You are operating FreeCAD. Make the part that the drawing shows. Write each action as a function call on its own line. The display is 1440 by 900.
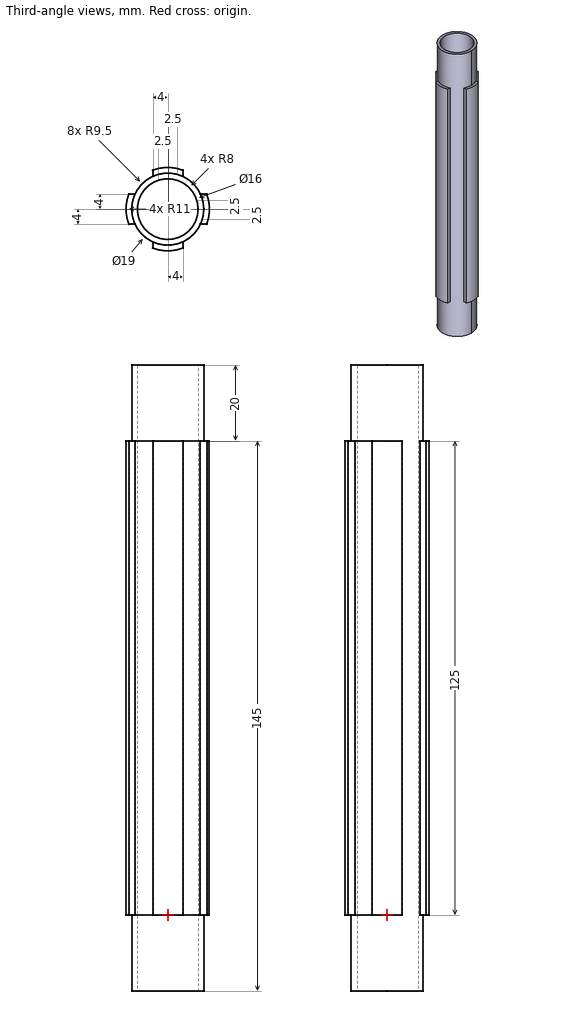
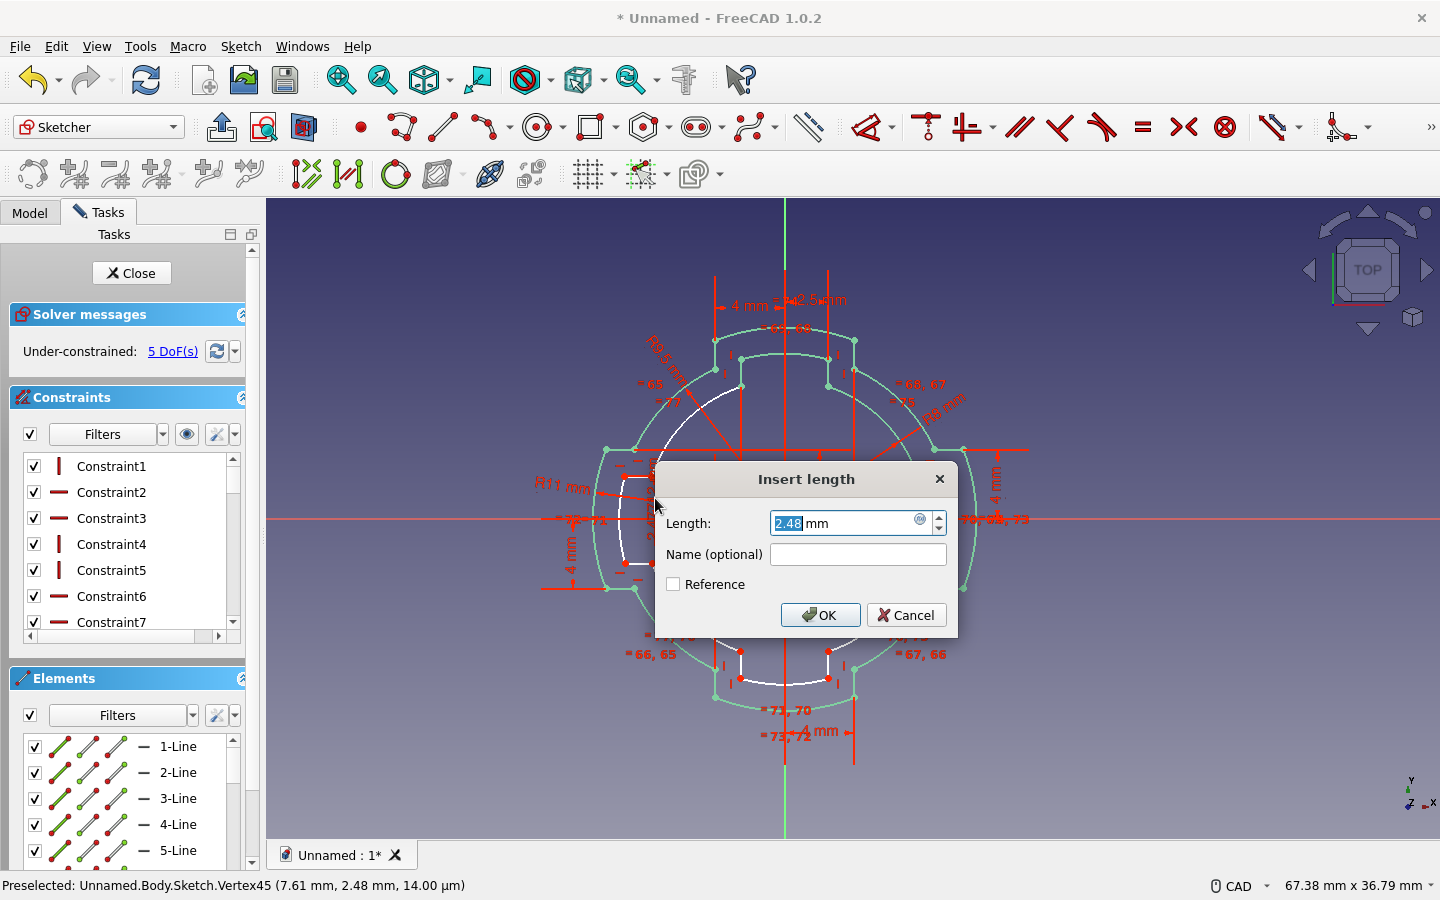
text(2.5)
key(Return)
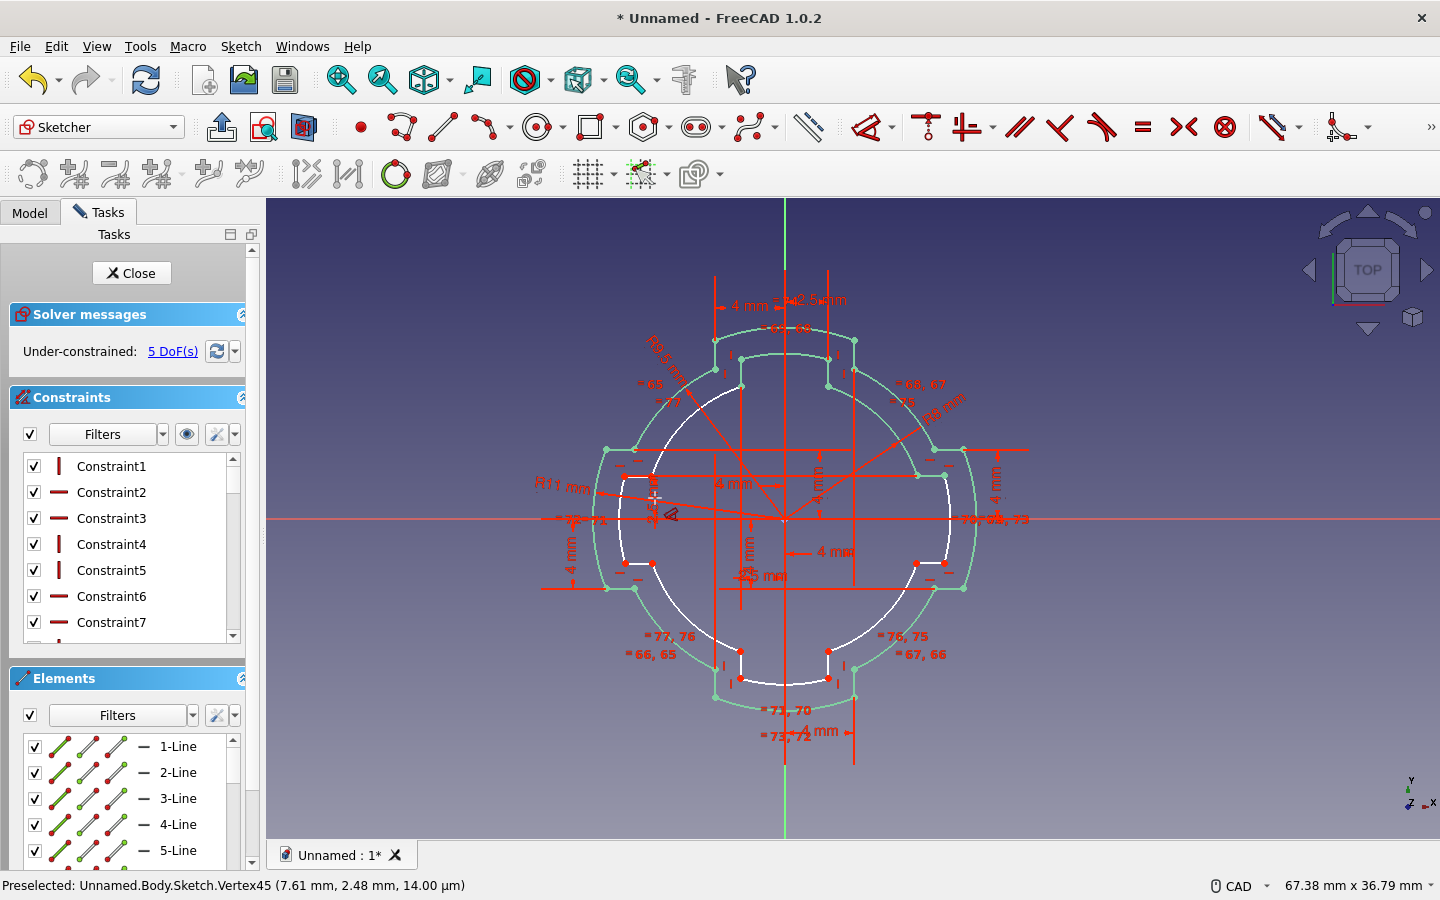
click(944, 563)
click(1002, 541)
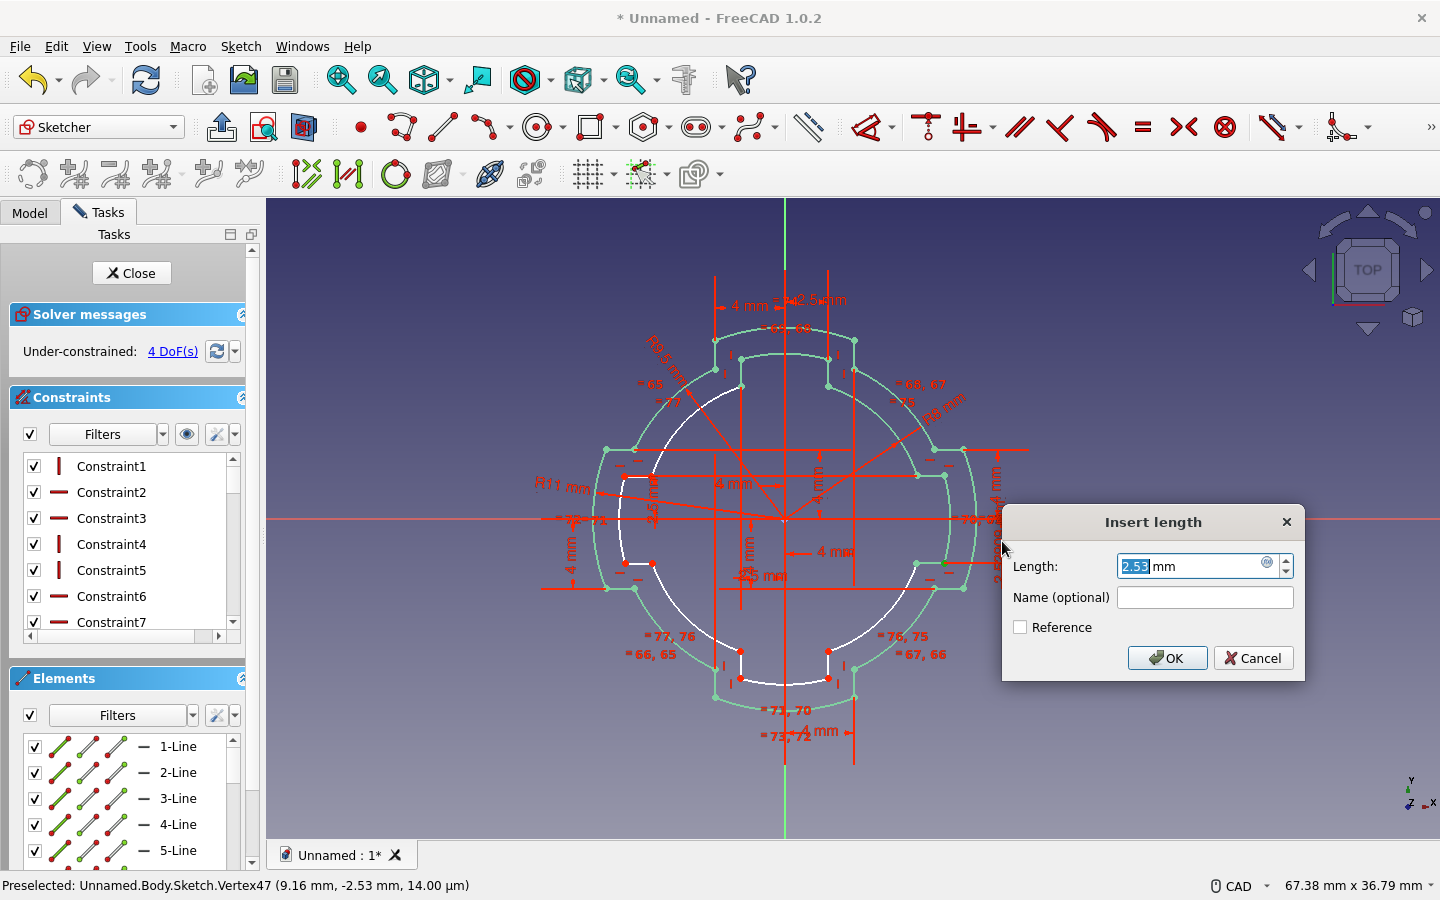
text(2.5)
key(Return)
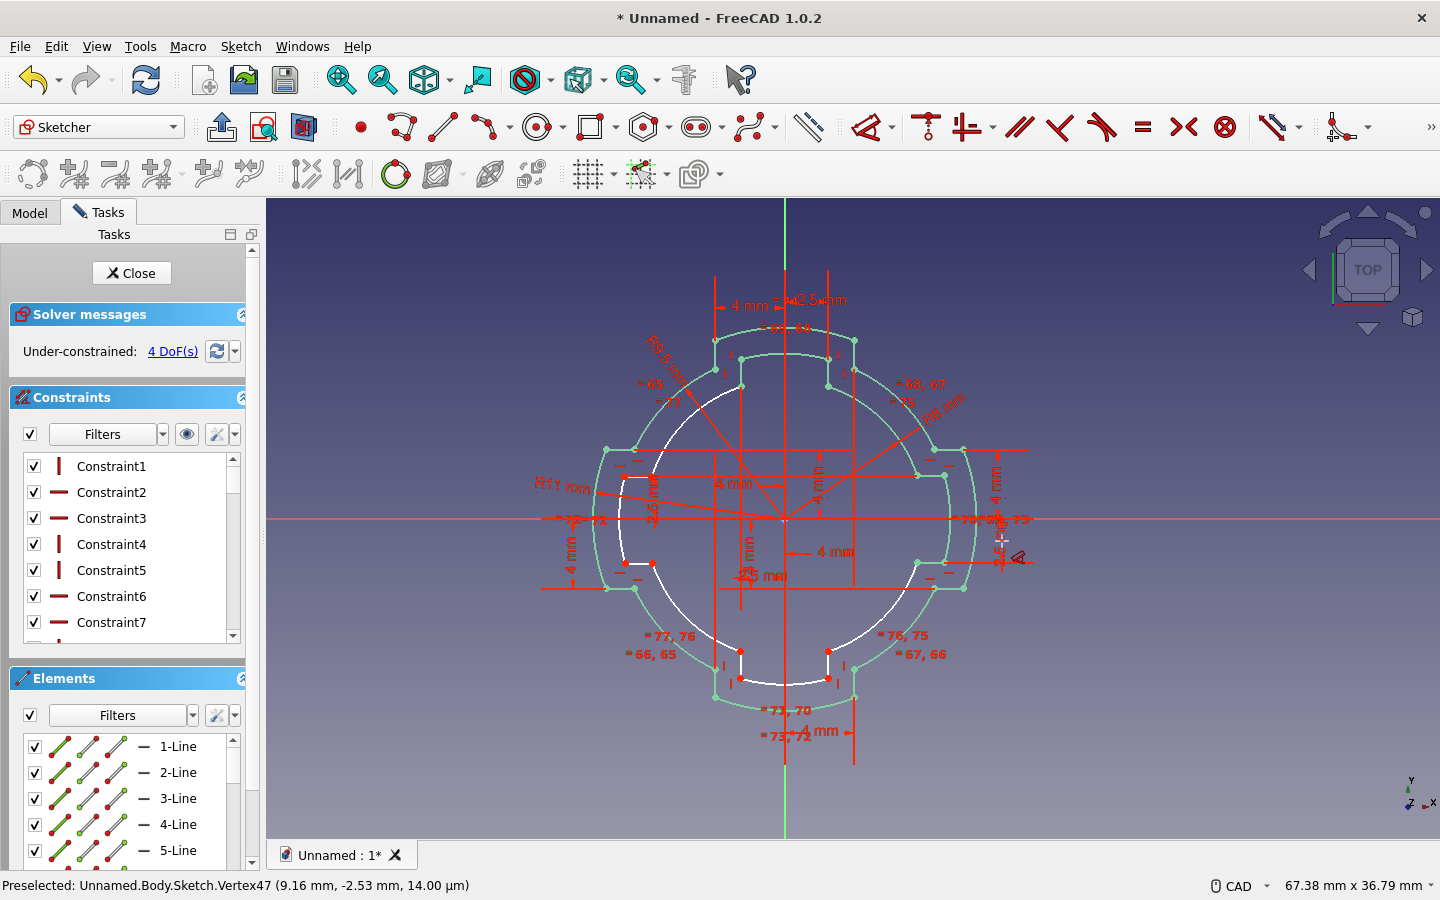
click(828, 652)
click(806, 461)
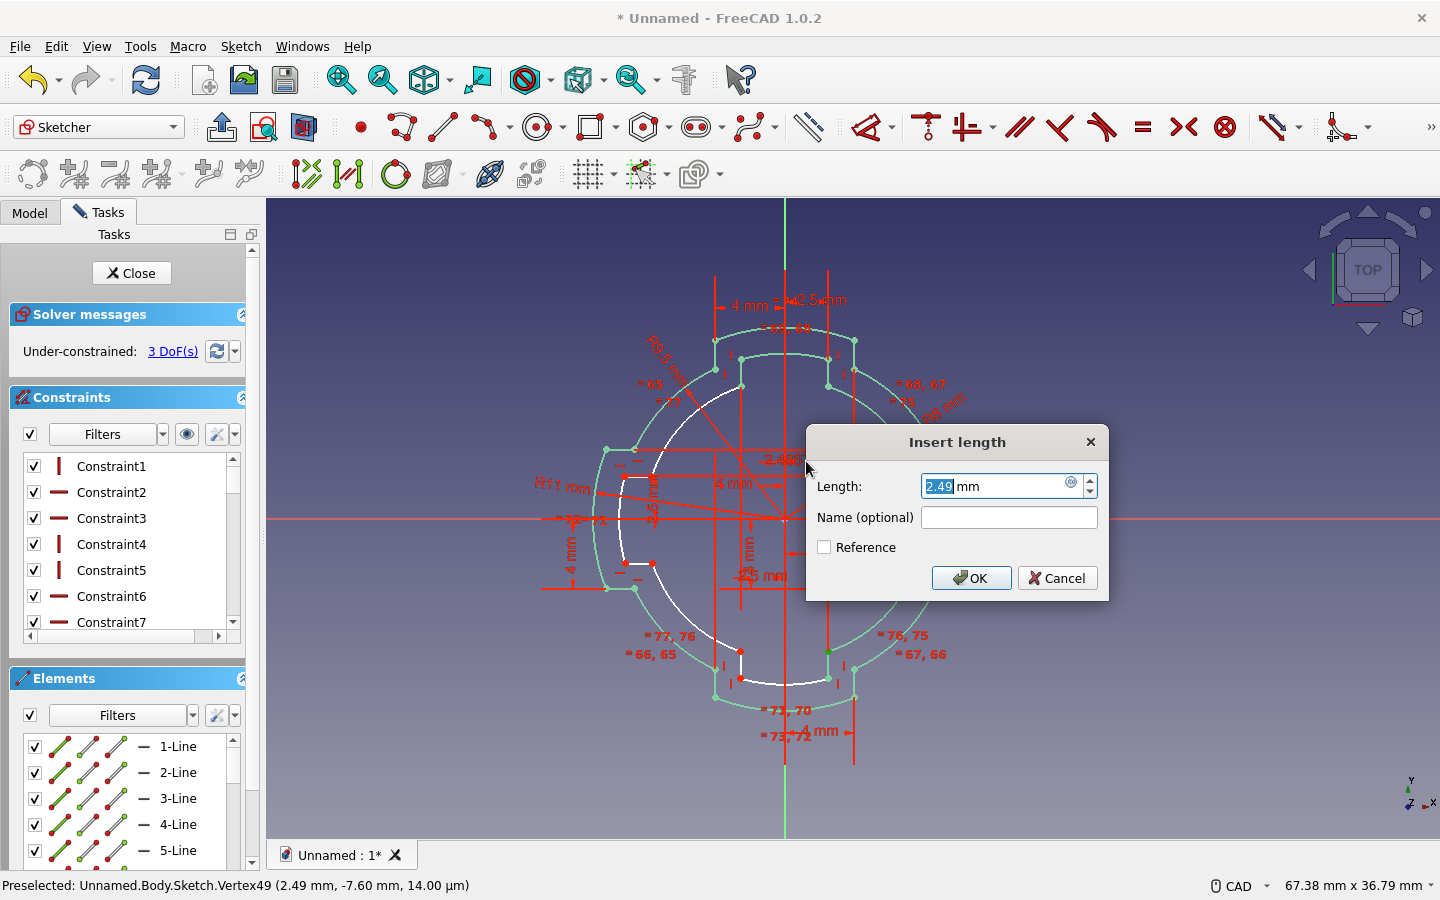
text(2.5)
key(Return)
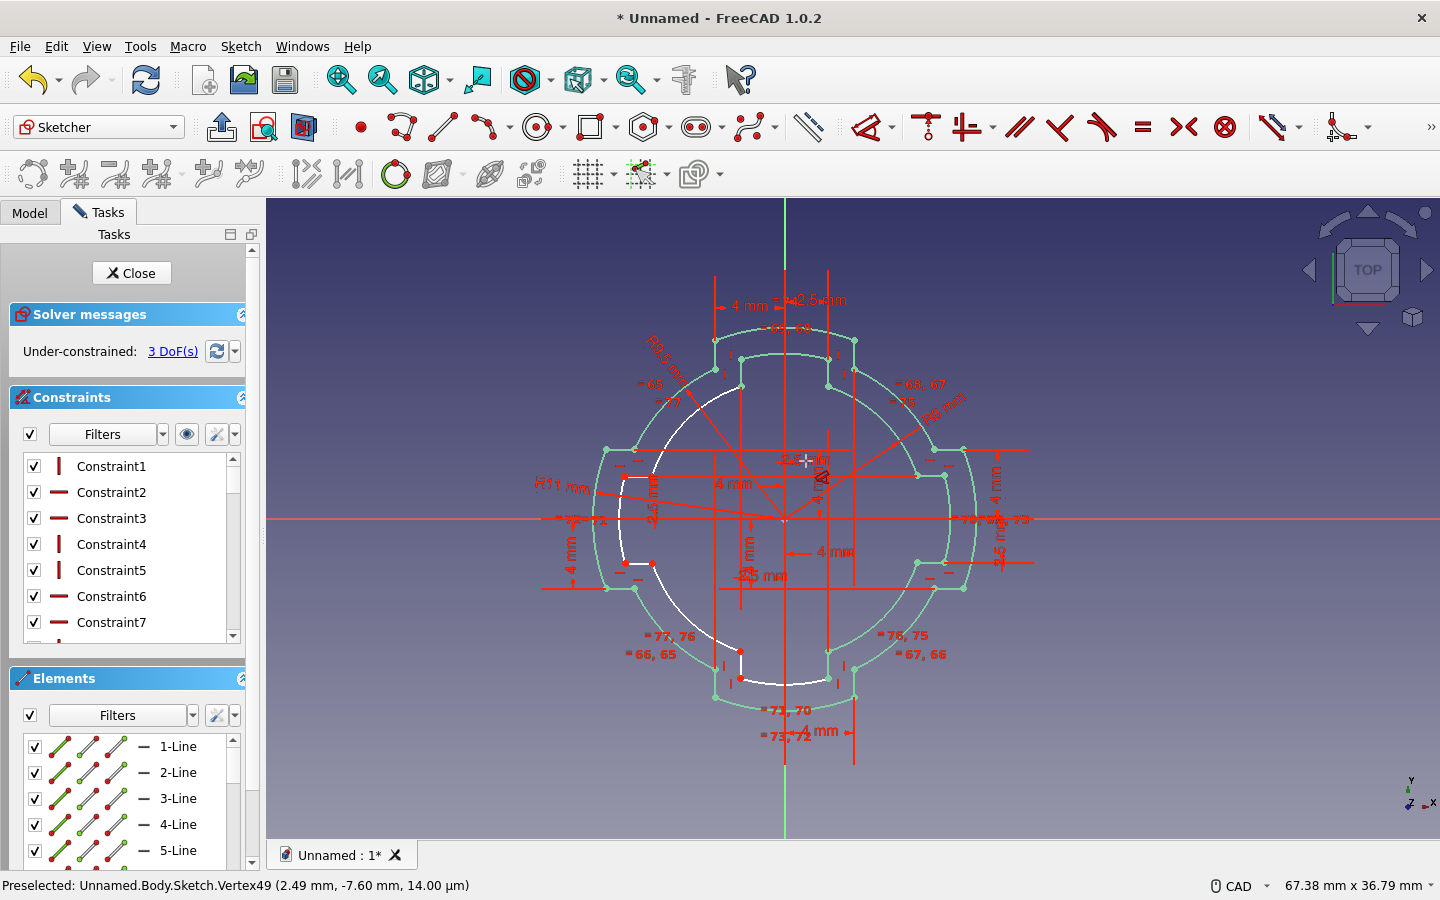
click(741, 679)
click(747, 737)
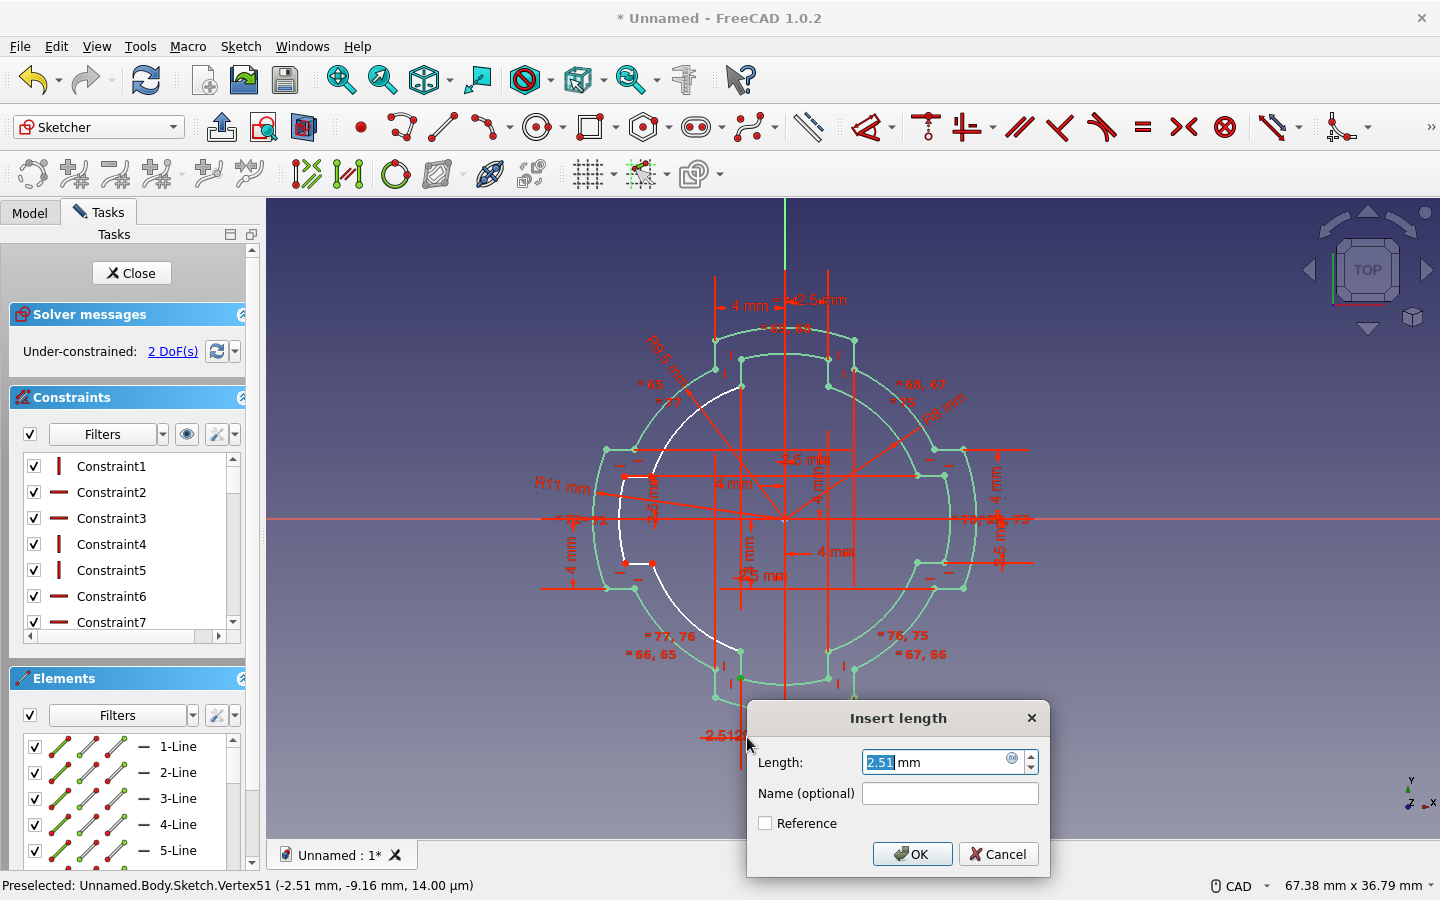
text(2.5)
key(Return)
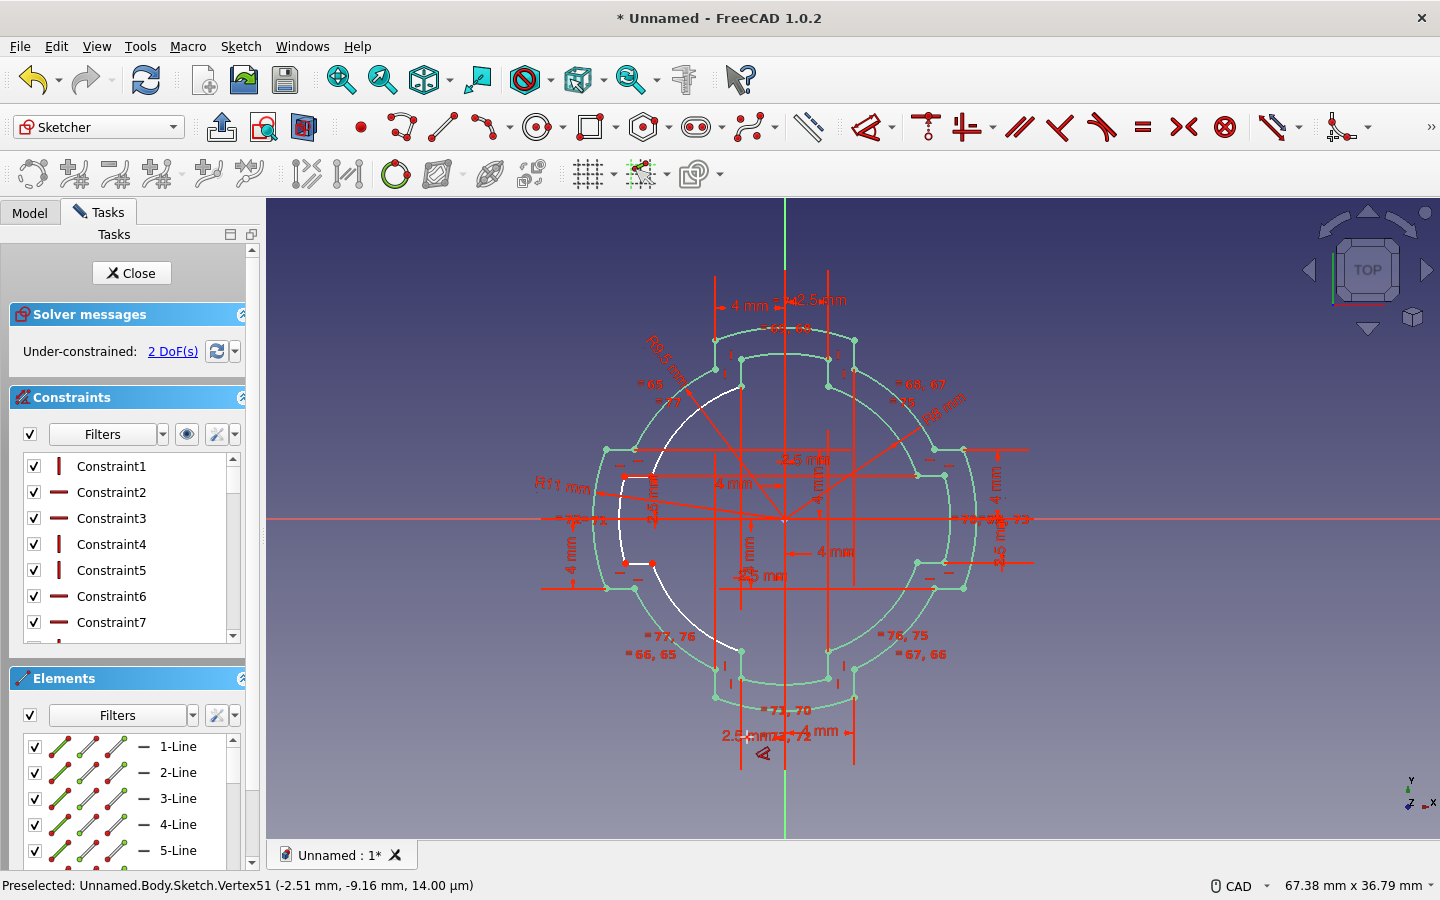
click(653, 564)
click(915, 542)